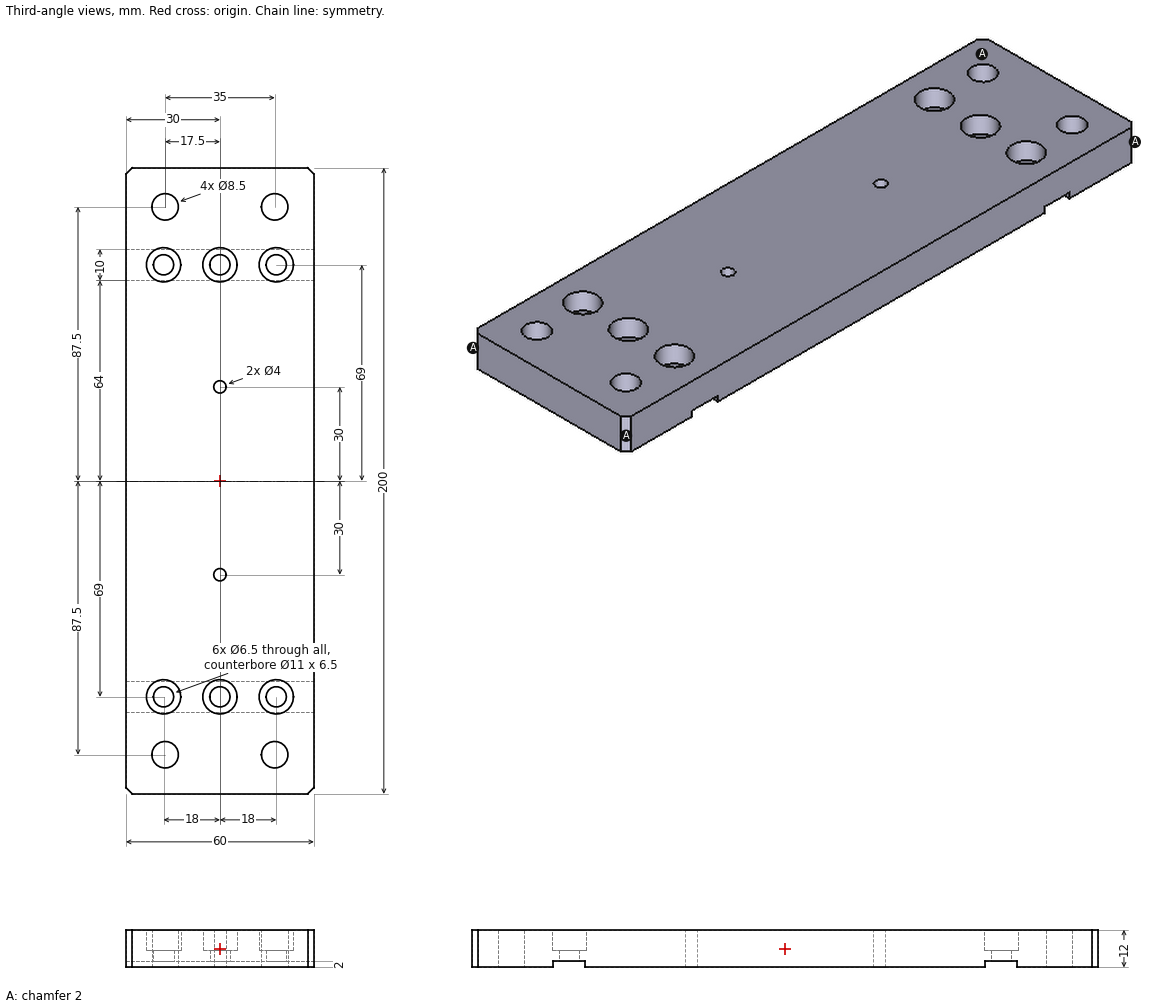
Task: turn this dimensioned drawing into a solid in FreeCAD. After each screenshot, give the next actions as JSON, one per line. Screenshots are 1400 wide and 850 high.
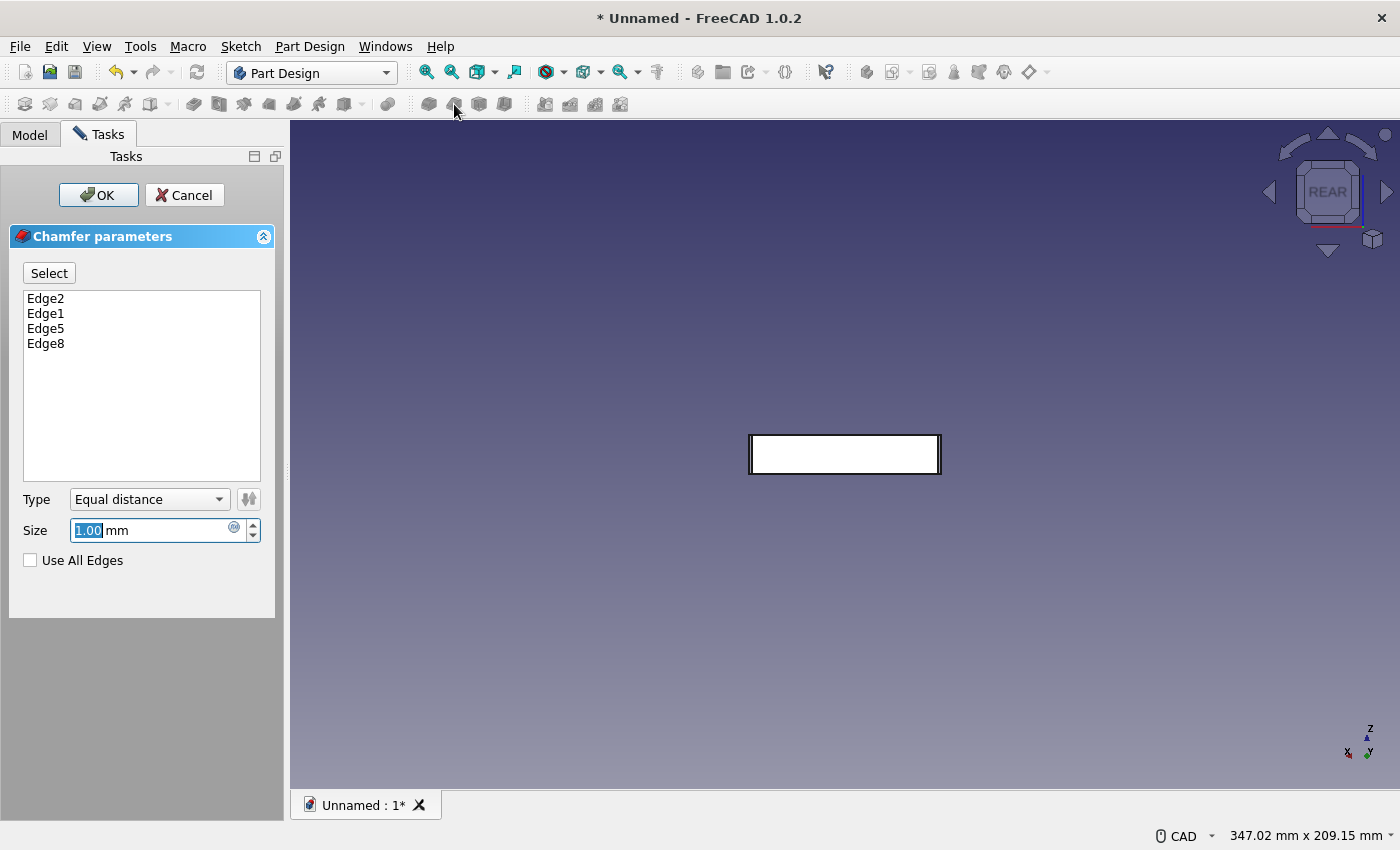
{"action": "type", "text": "2"}
{"action": "key", "text": "Tab"}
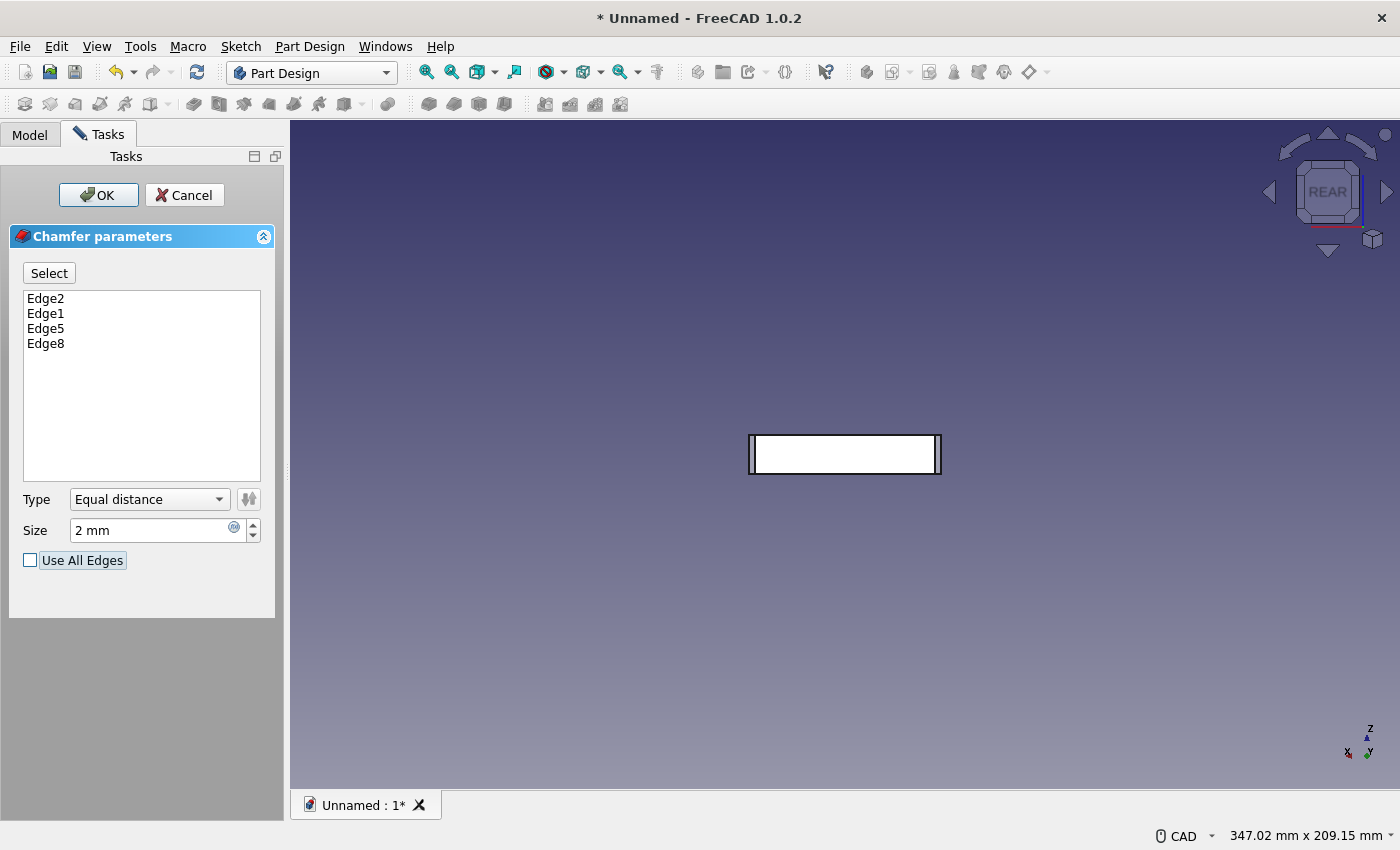
{"action": "left_click", "coordinate": [99, 195]}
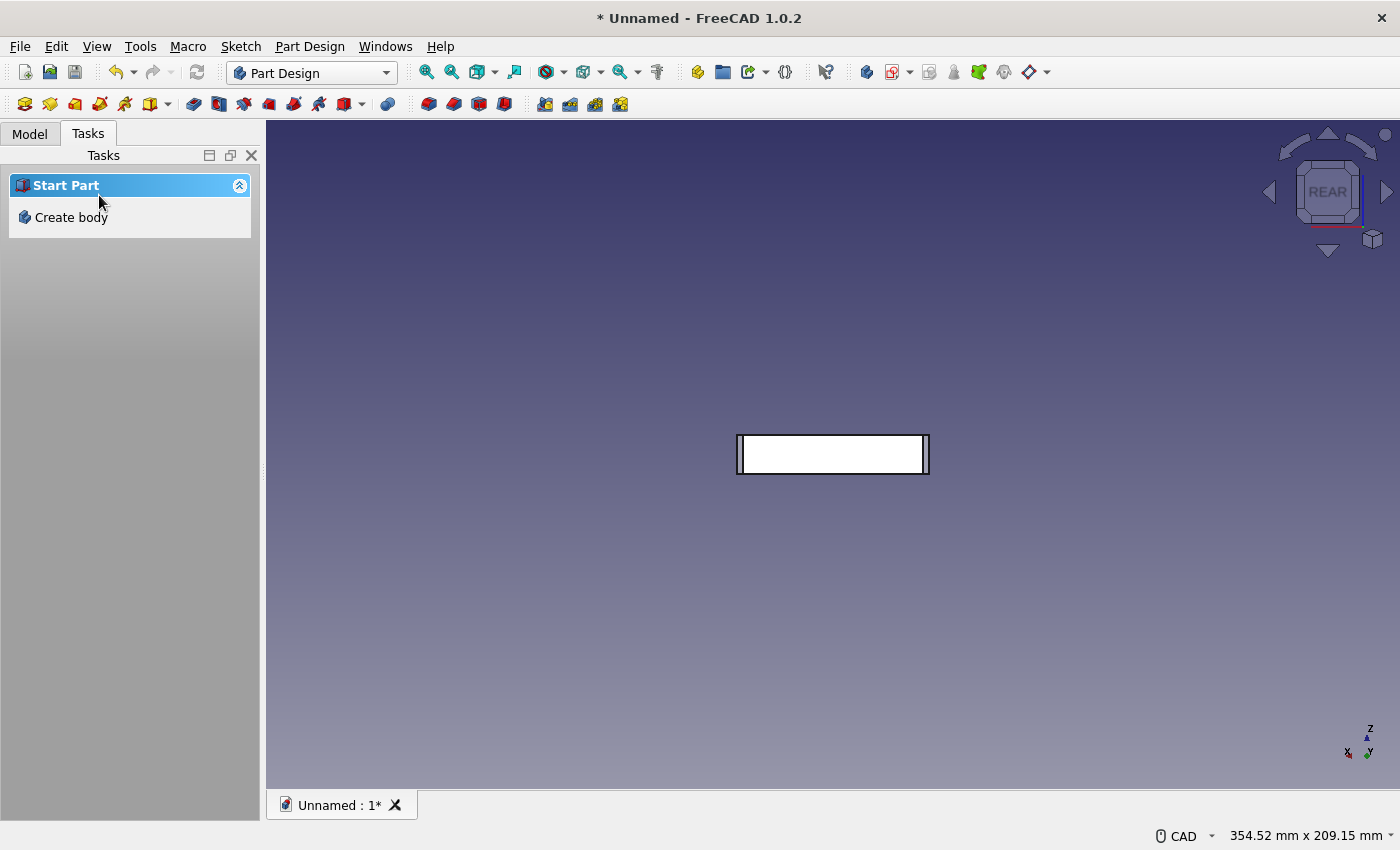
{"action": "left_click", "coordinate": [427, 72]}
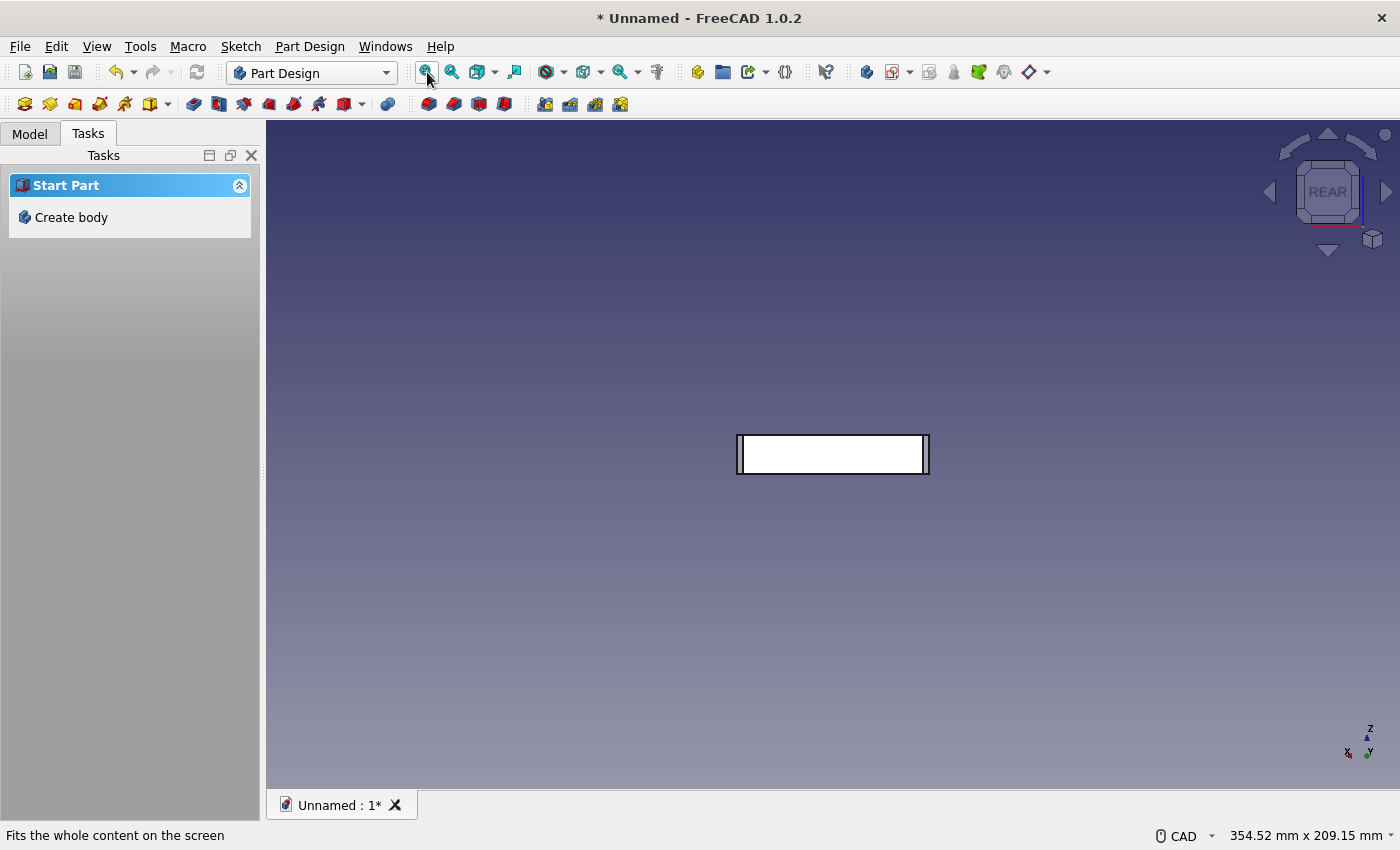
{"action": "key", "text": "5"}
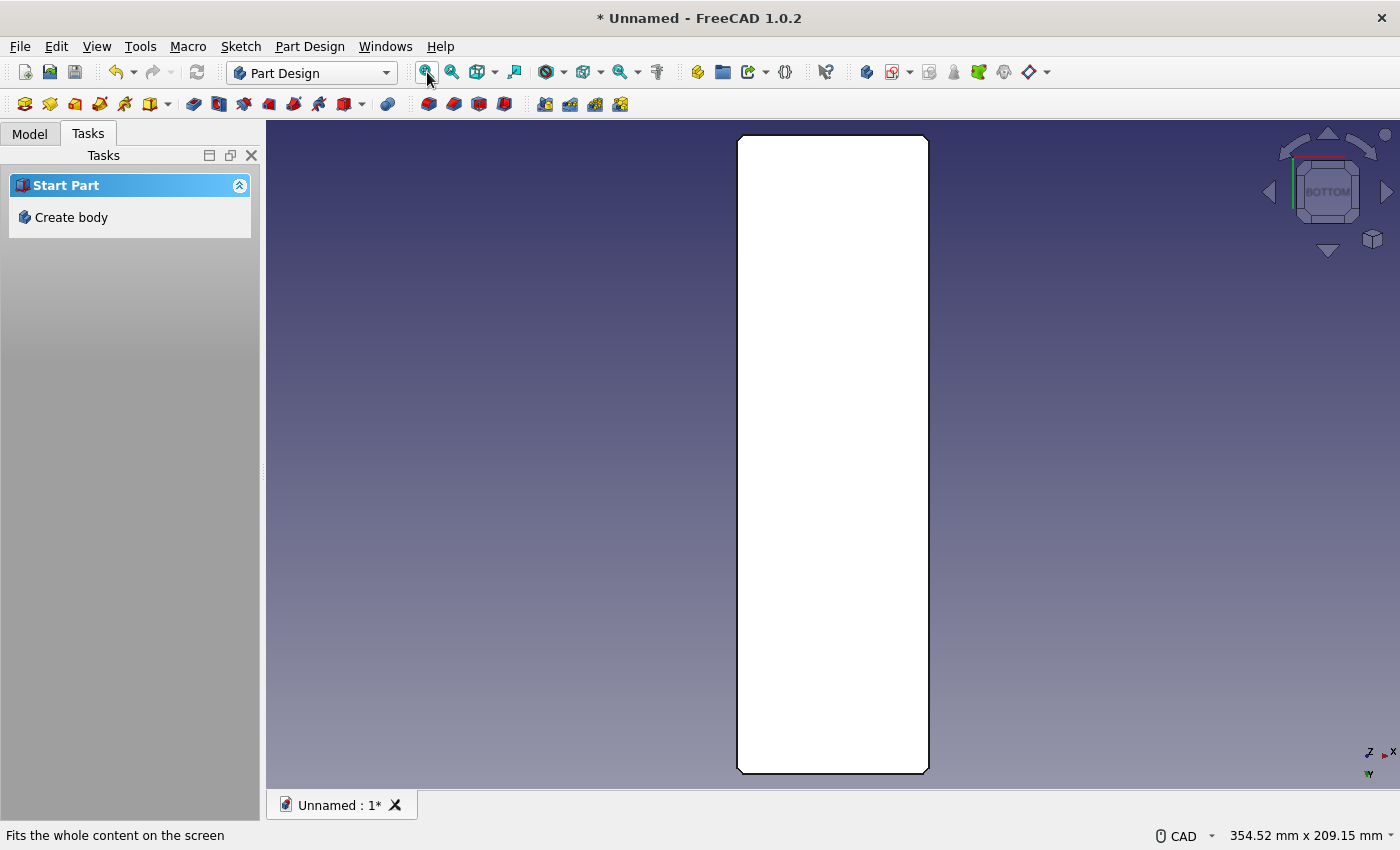
{"action": "left_click", "coordinate": [833, 636]}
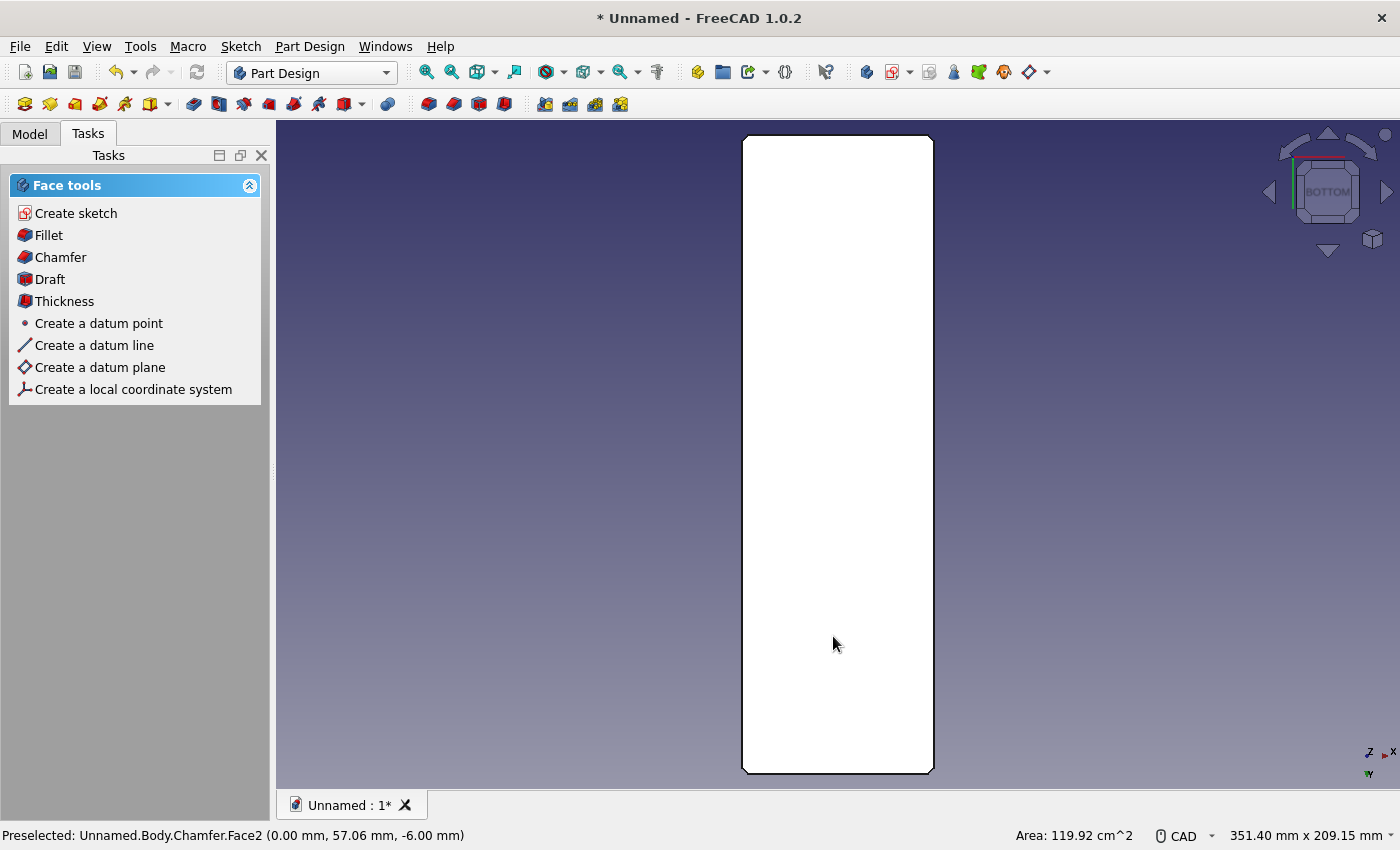
{"action": "left_click", "coordinate": [892, 72]}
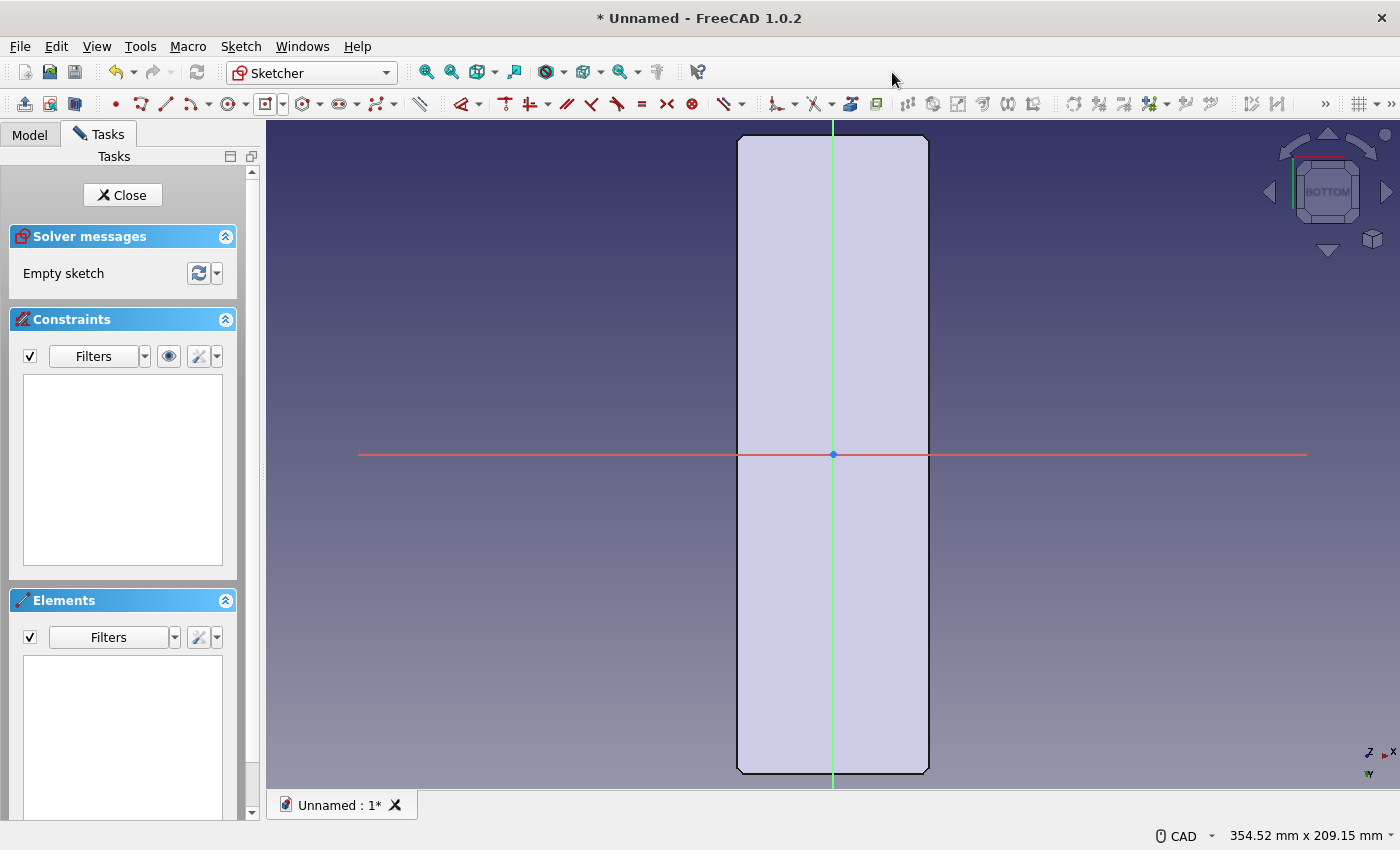
{"action": "left_click", "coordinate": [282, 104]}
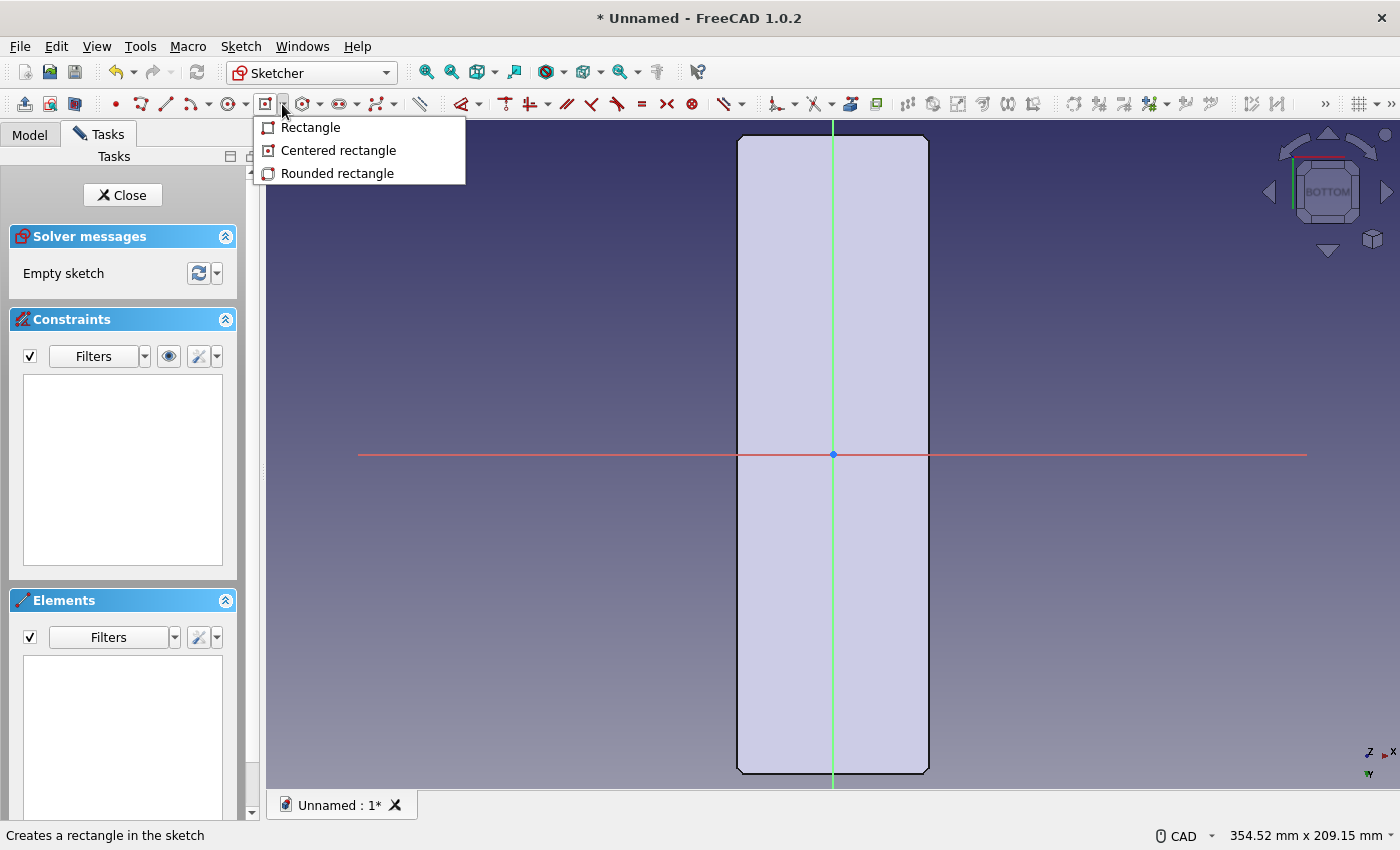
{"action": "left_click", "coordinate": [360, 128]}